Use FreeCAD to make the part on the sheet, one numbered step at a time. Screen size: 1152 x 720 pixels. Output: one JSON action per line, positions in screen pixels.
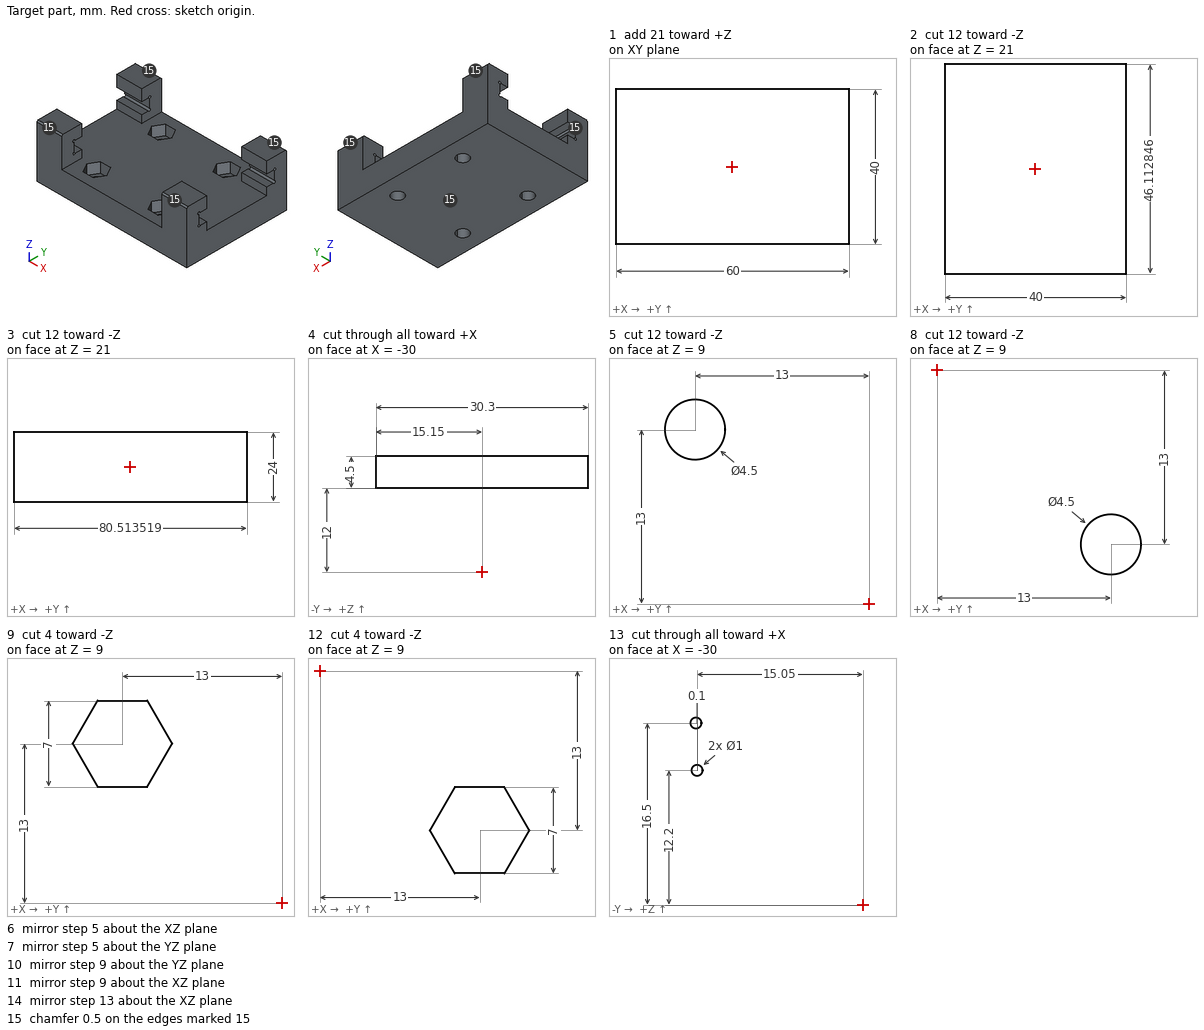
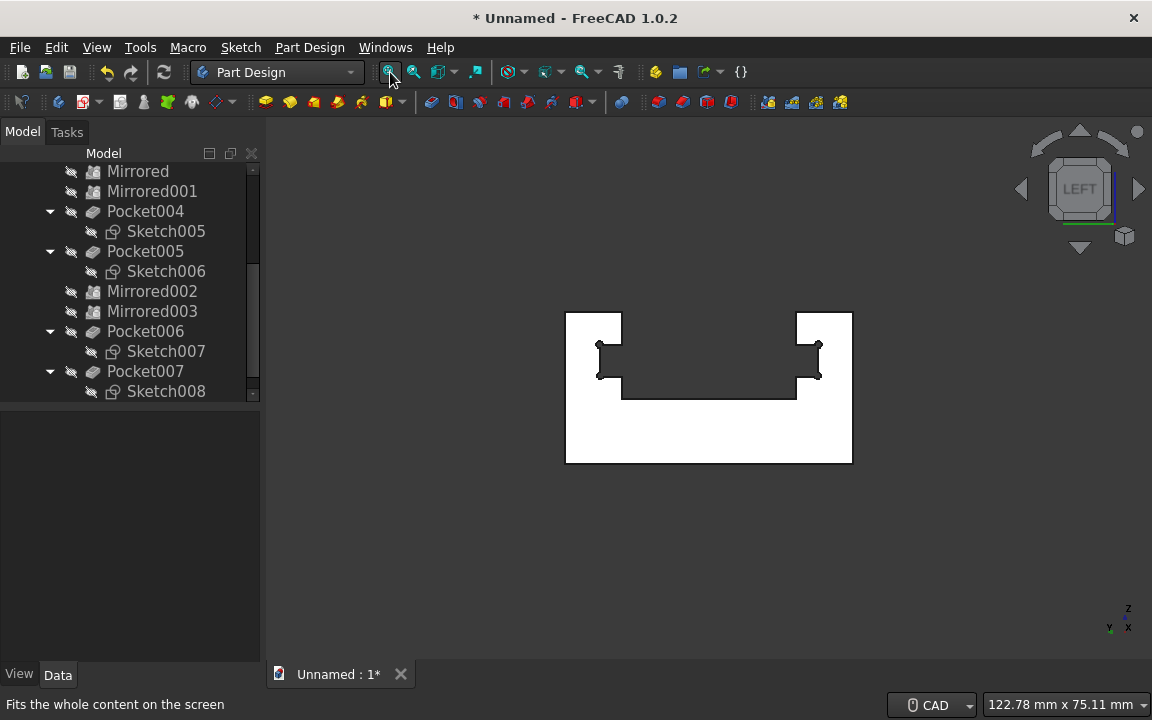
{"action": "key", "text": "0"}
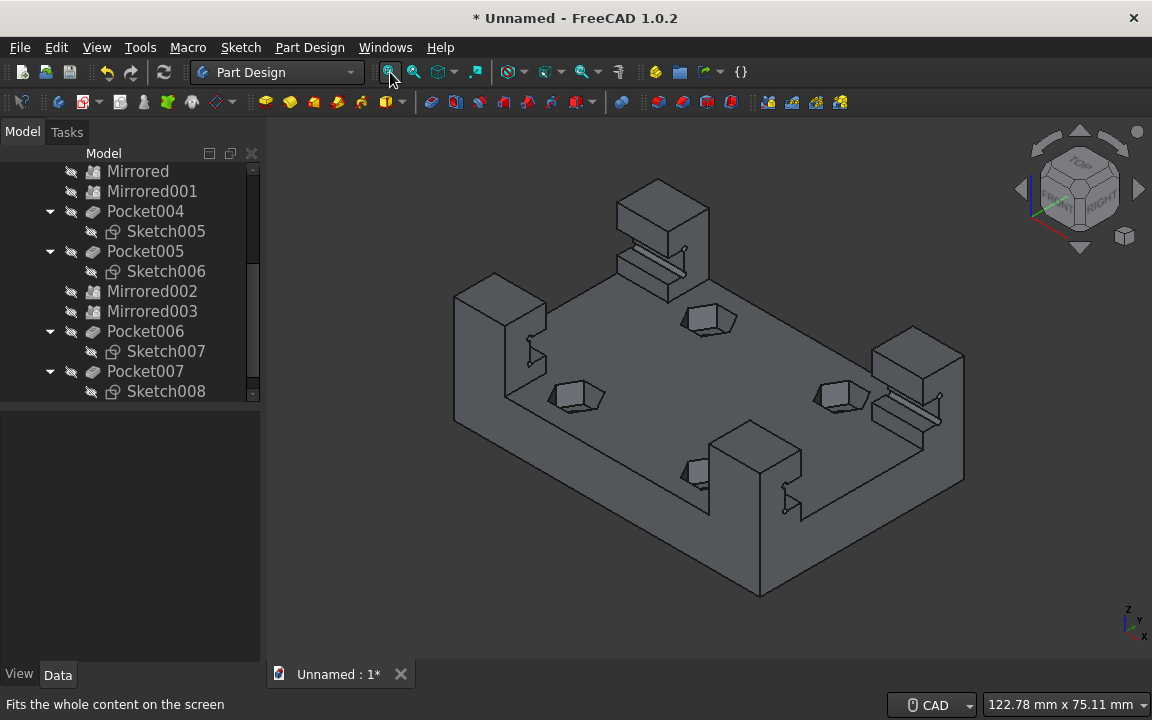
{"action": "left_click", "coordinate": [735, 458]}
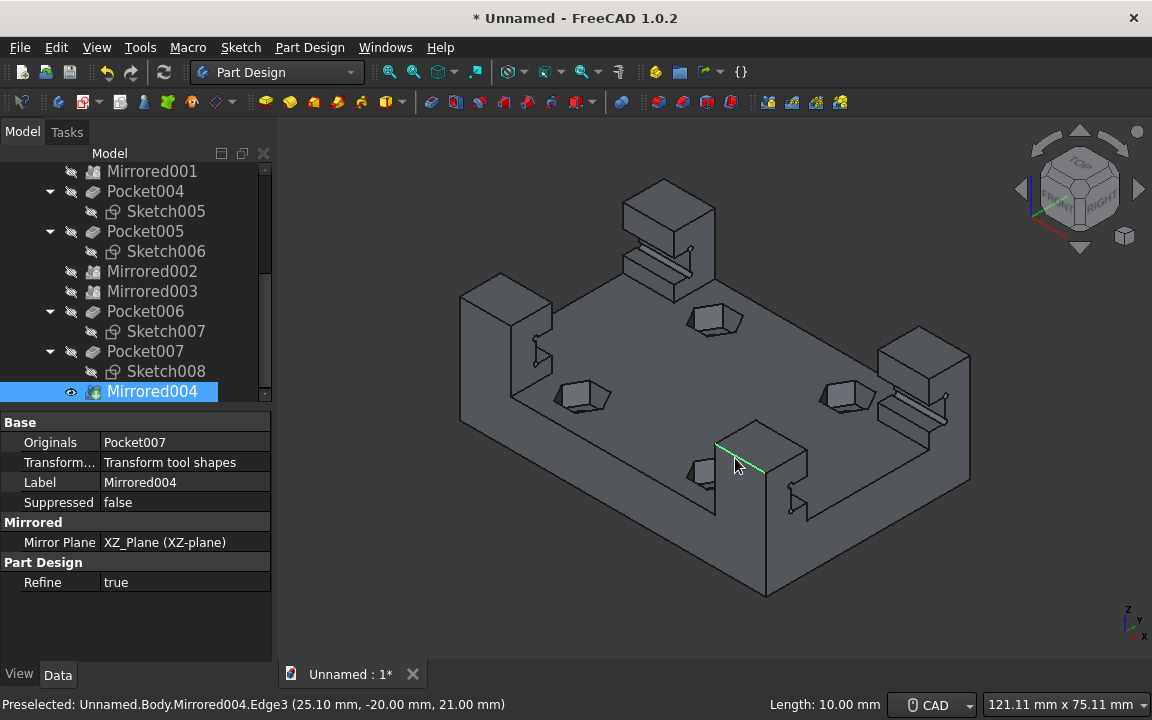
{"action": "left_click", "coordinate": [485, 310], "text": "ctrl"}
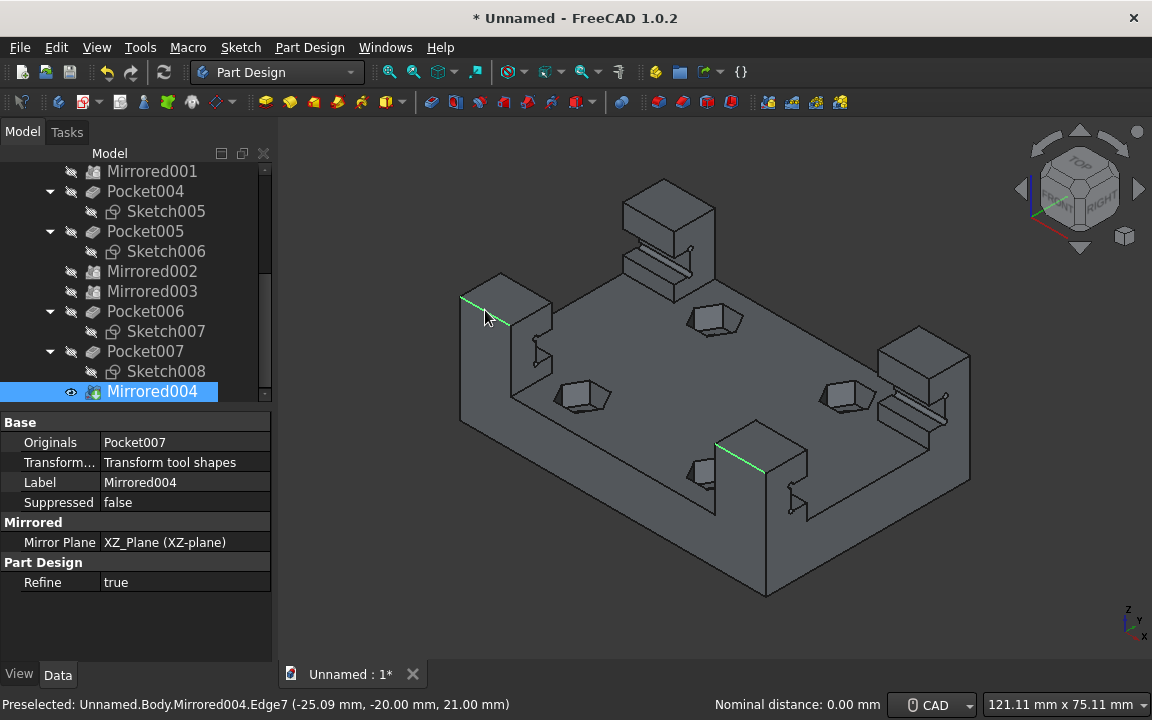
{"action": "key", "text": "2"}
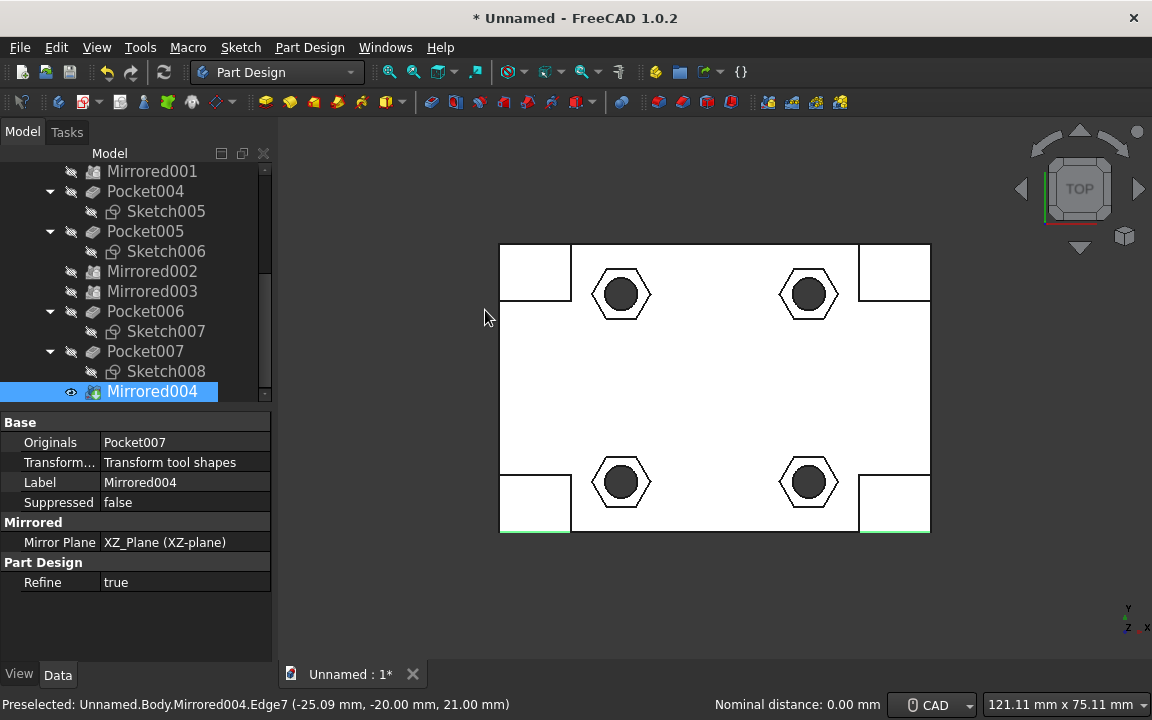
{"action": "left_click", "coordinate": [535, 243], "text": "ctrl"}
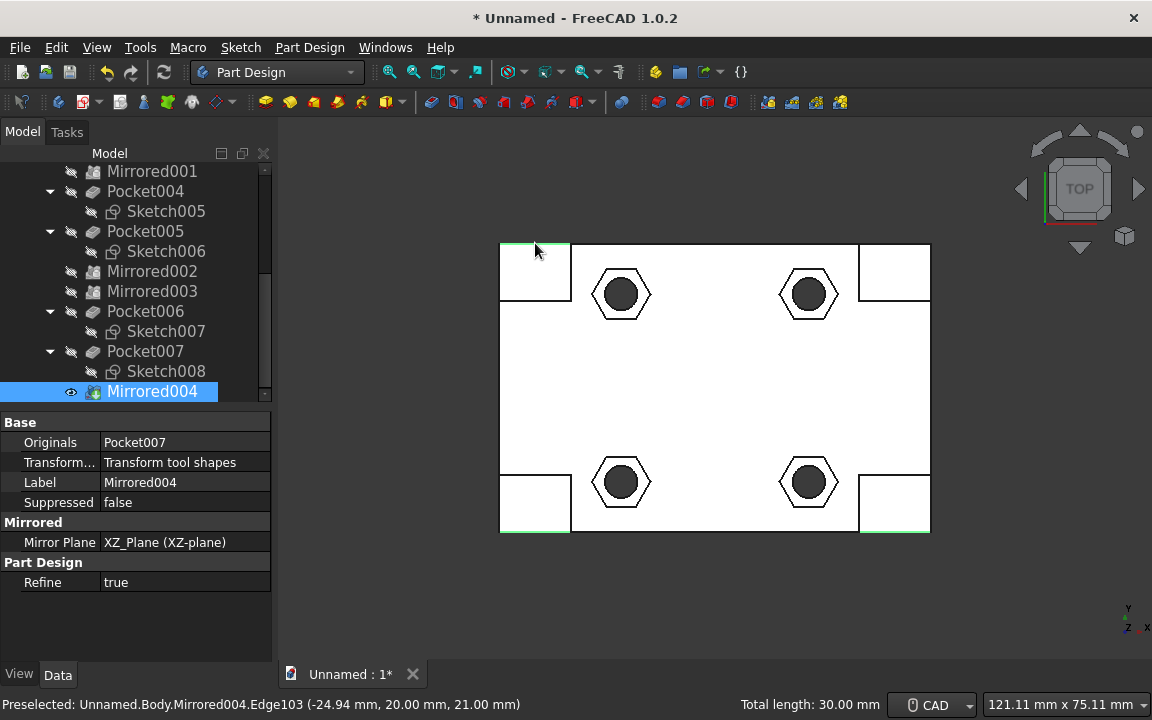
{"action": "left_click", "coordinate": [895, 243], "text": "ctrl"}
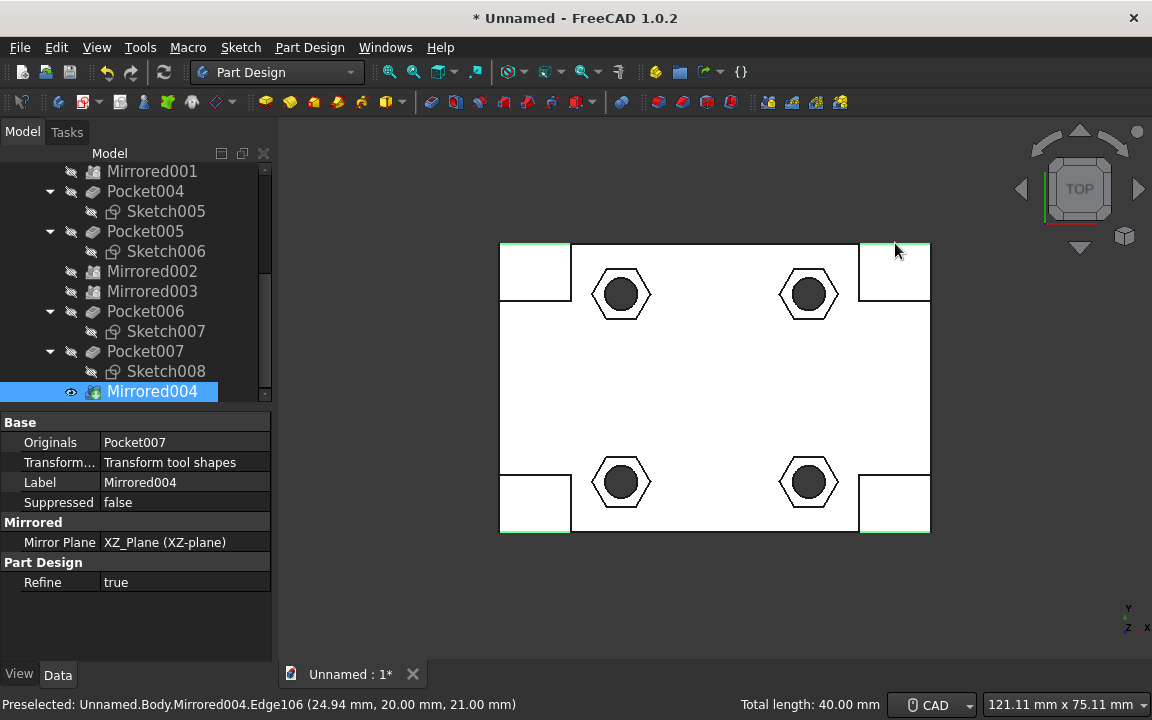
{"action": "left_click", "coordinate": [684, 102]}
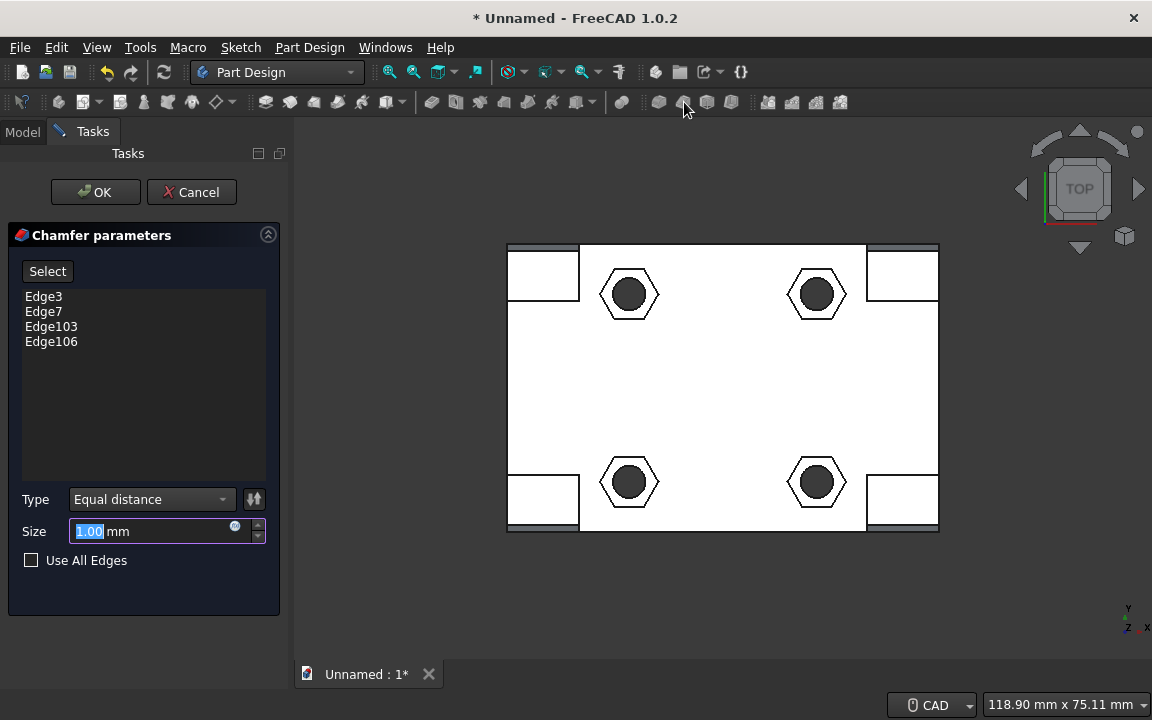
{"action": "type", "text": "0.5"}
{"action": "key", "text": "Tab"}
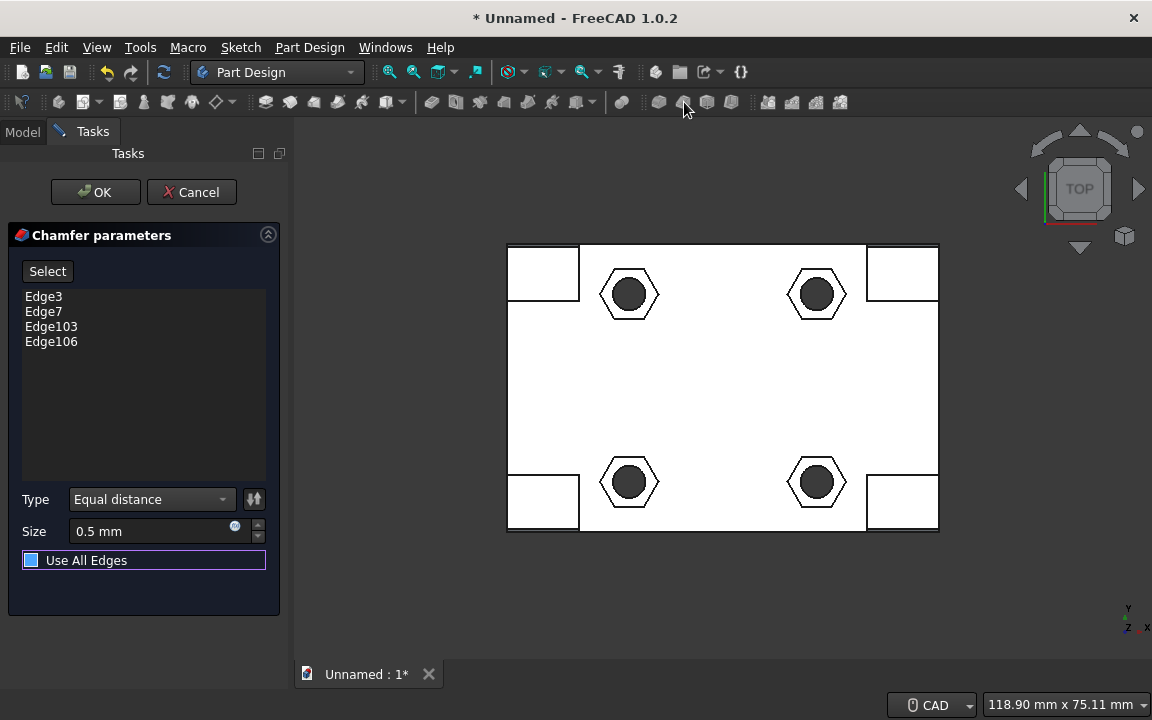
{"action": "left_click", "coordinate": [96, 192]}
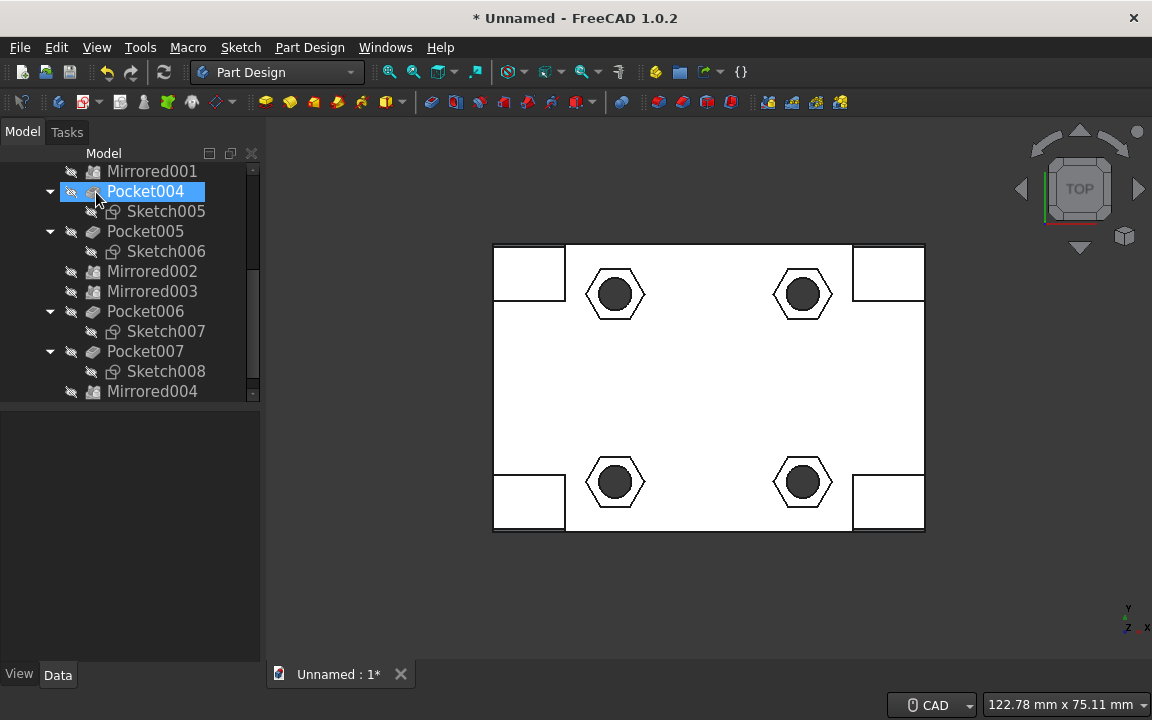
{"action": "key", "text": "0"}